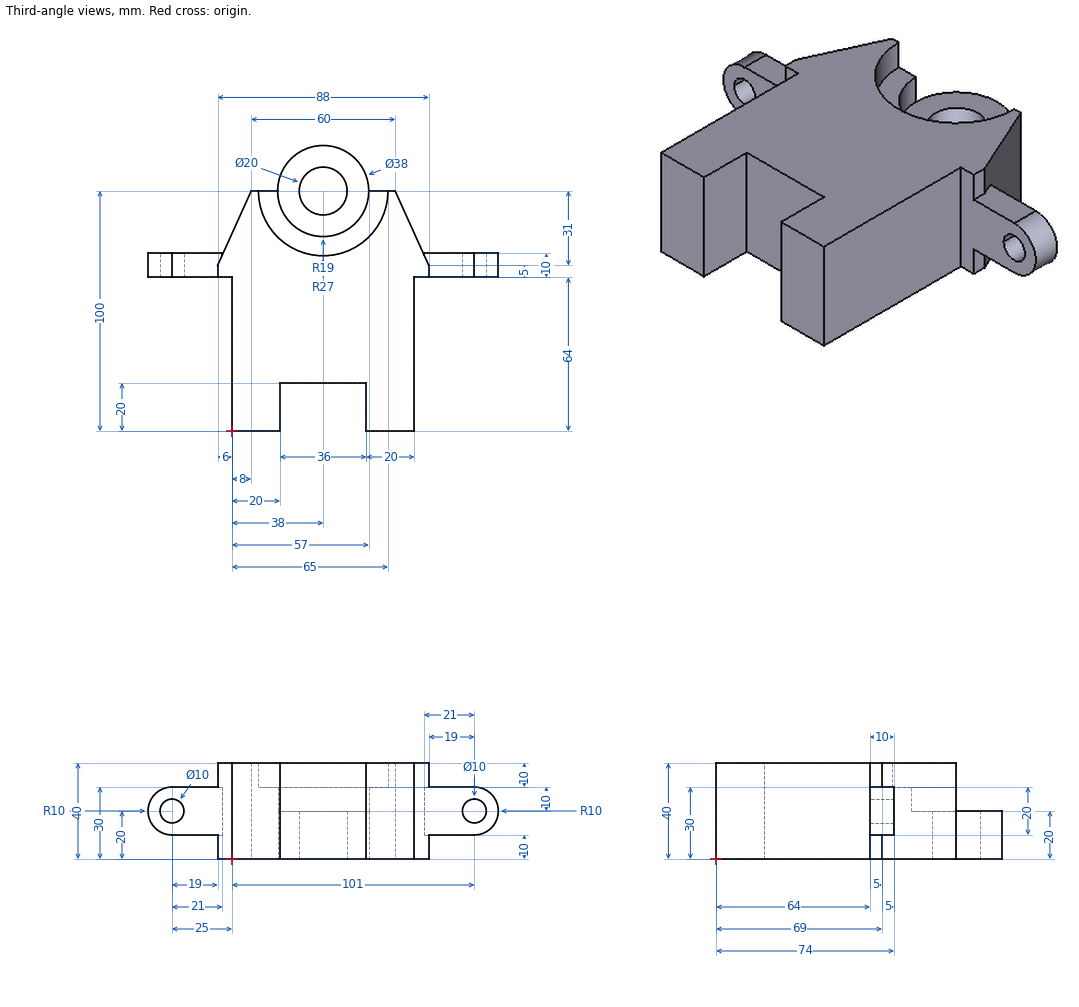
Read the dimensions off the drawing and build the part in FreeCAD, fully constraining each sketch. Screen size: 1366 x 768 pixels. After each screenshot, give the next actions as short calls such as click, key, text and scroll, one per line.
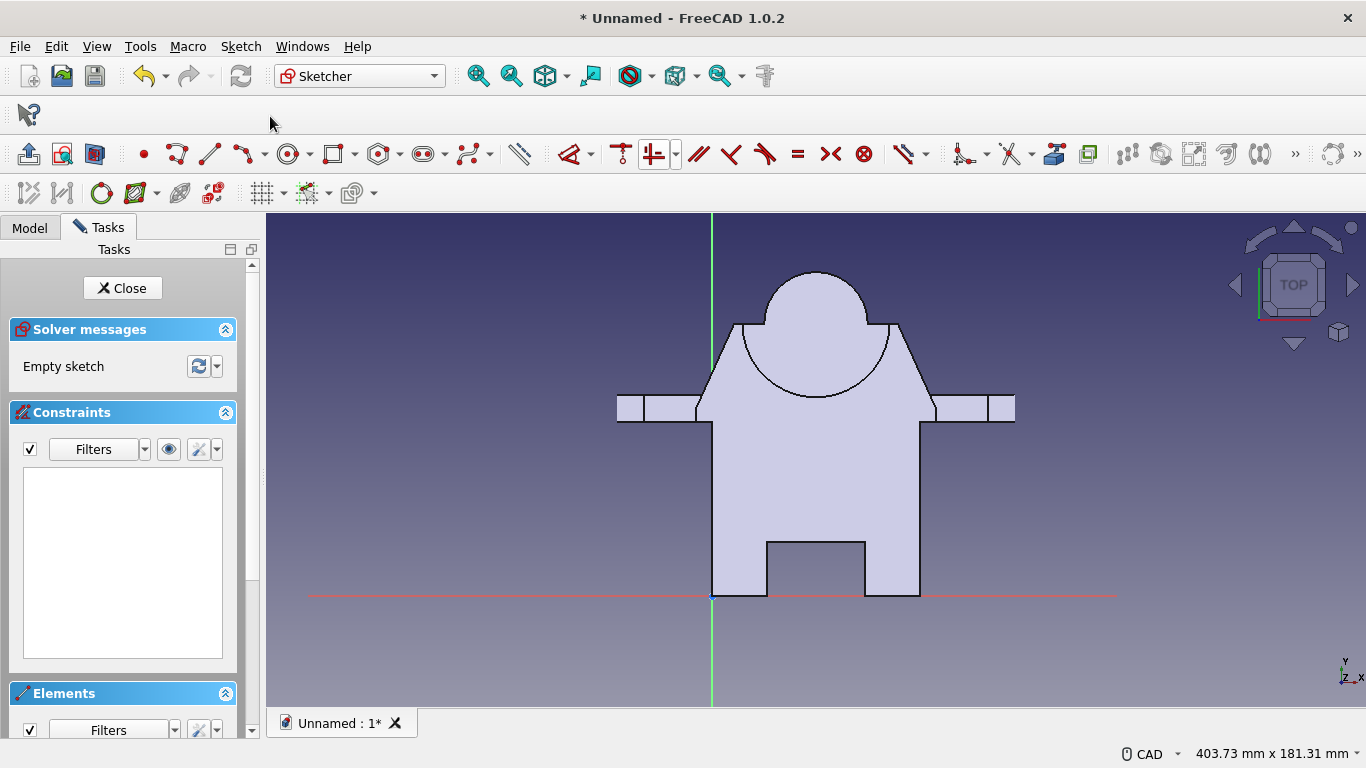
scroll(856, 244, up, 5)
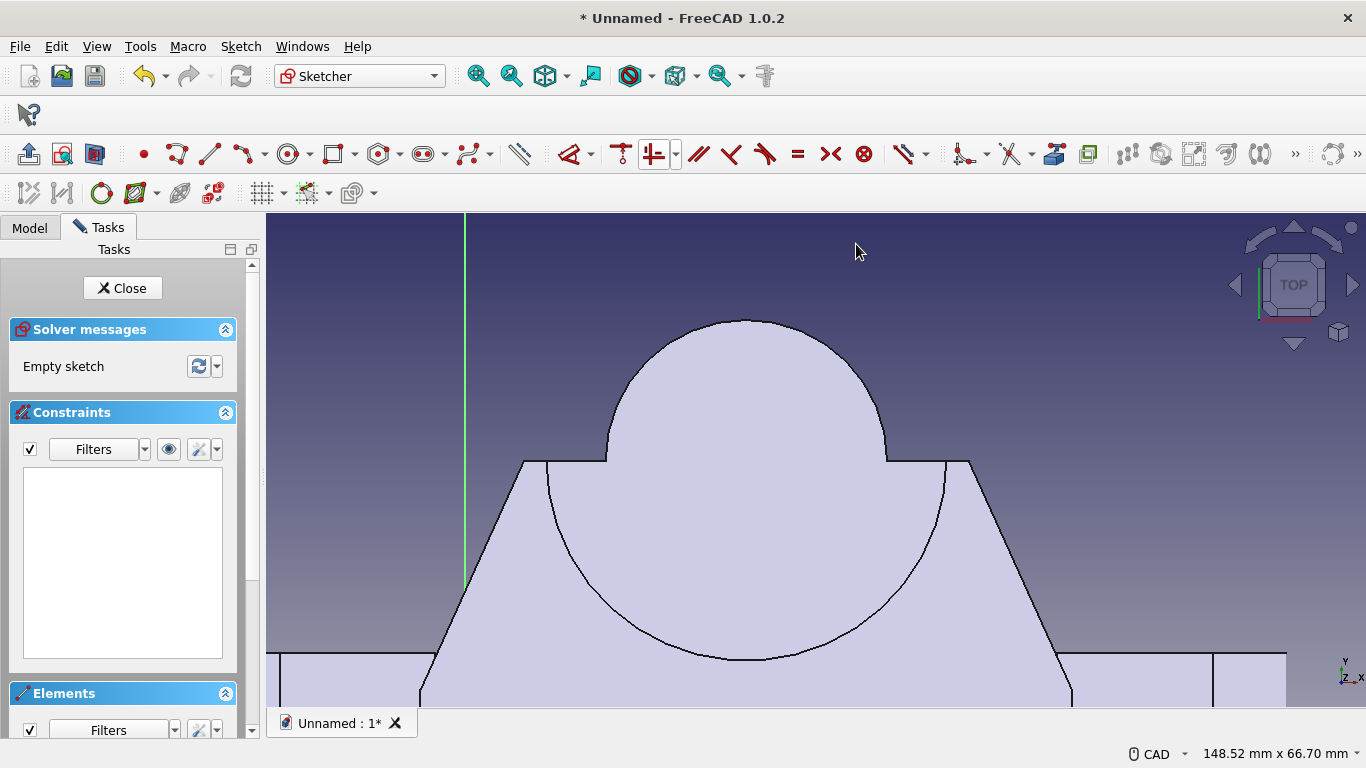
click(288, 154)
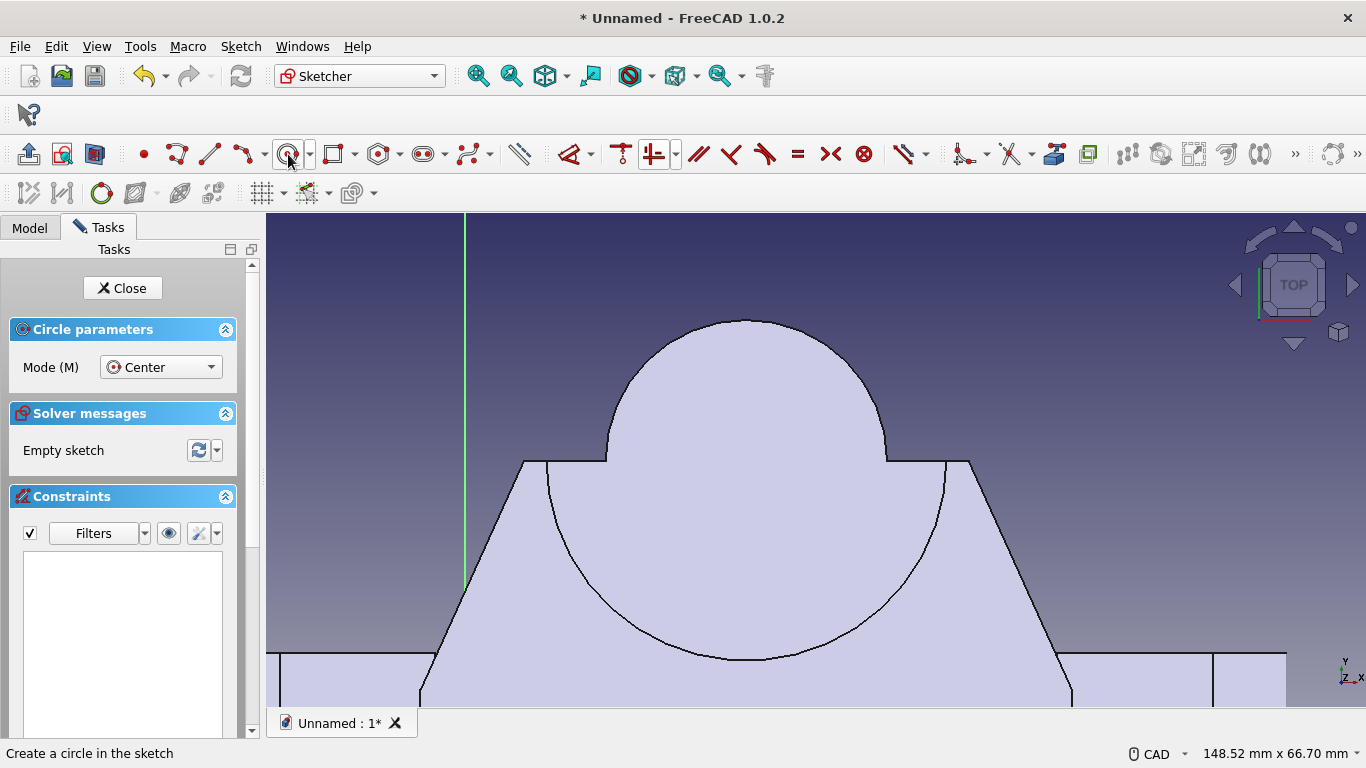
click(746, 461)
click(846, 361)
key(Escape)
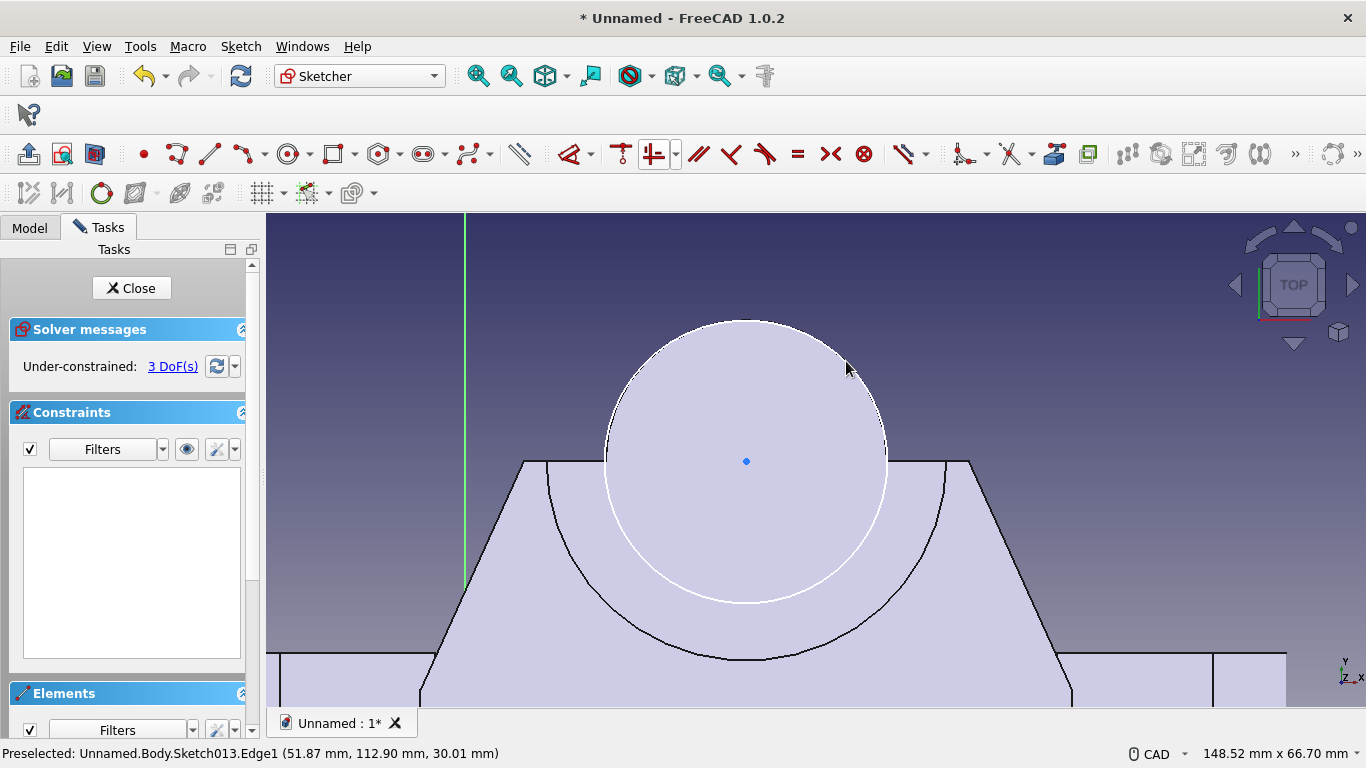
click(568, 154)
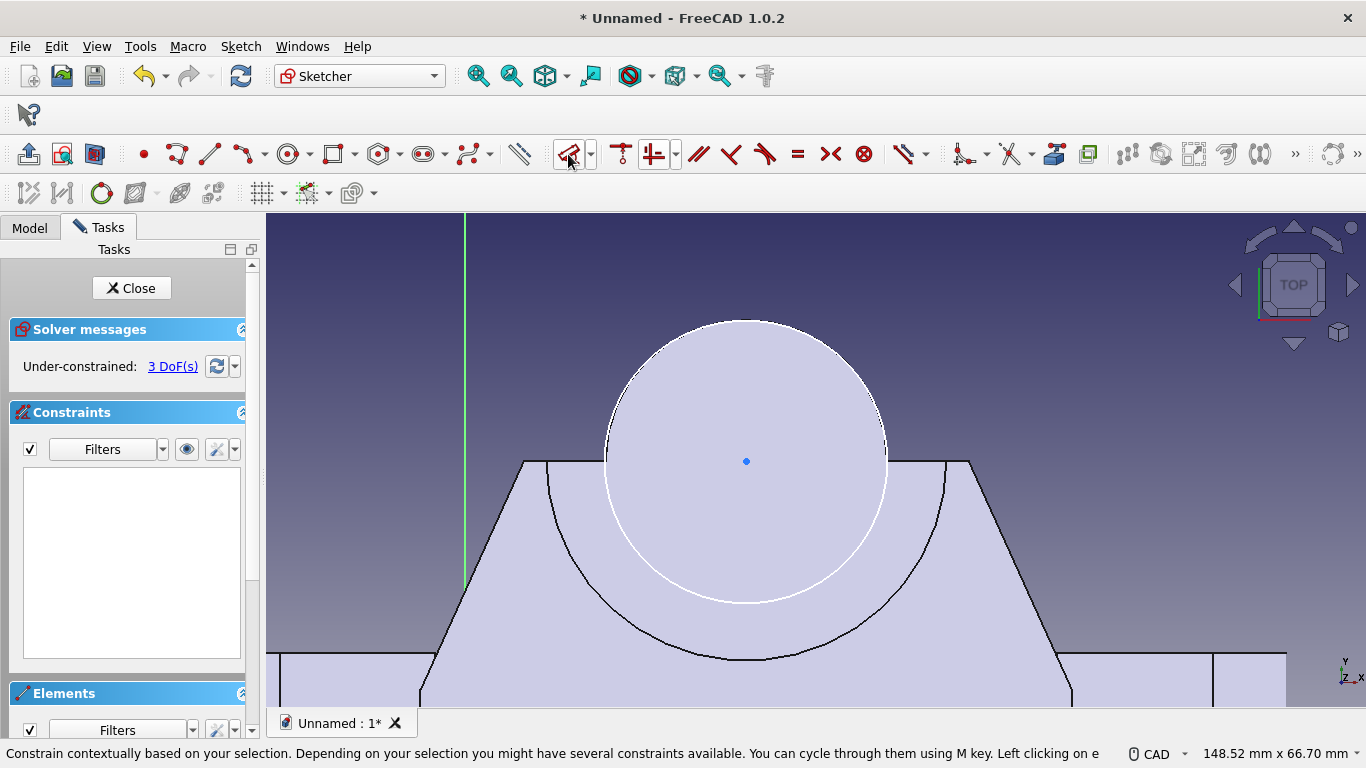
click(846, 362)
click(869, 339)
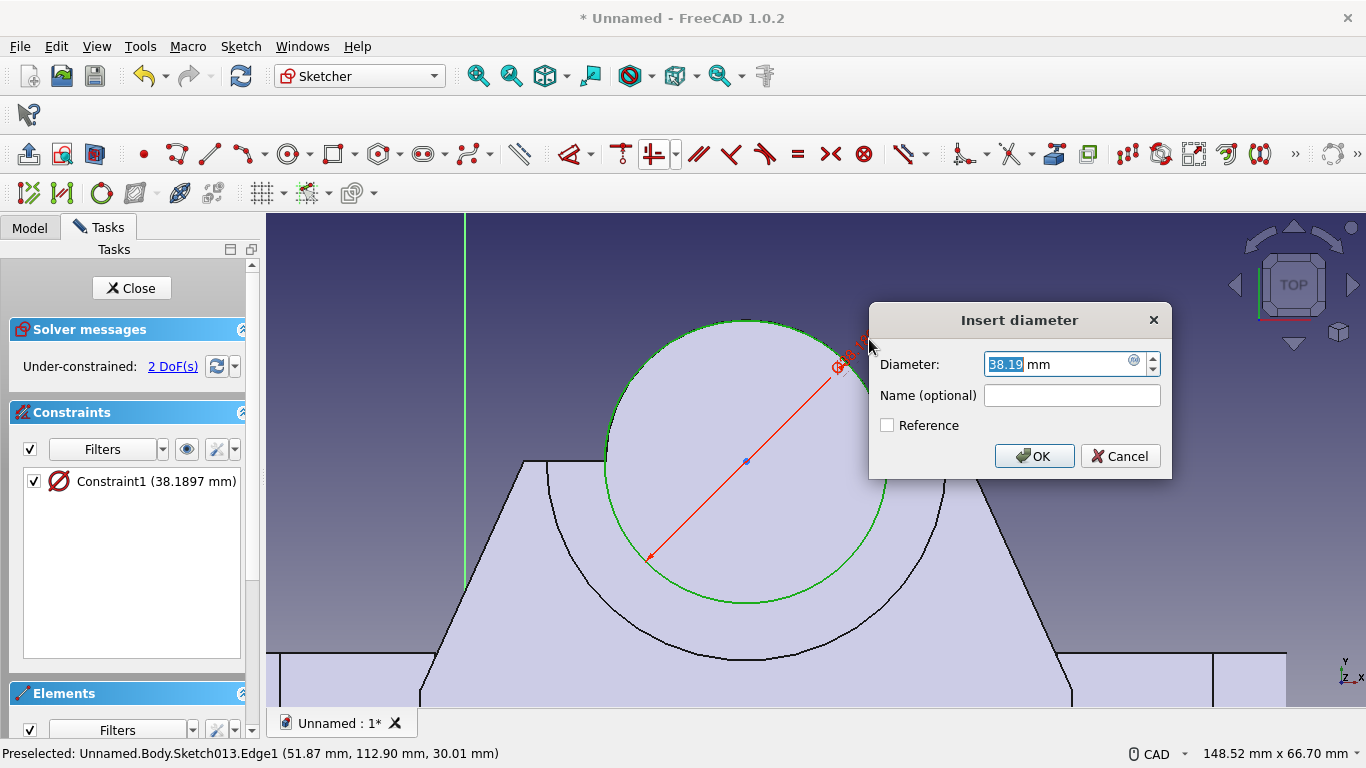
text(38)
key(Return)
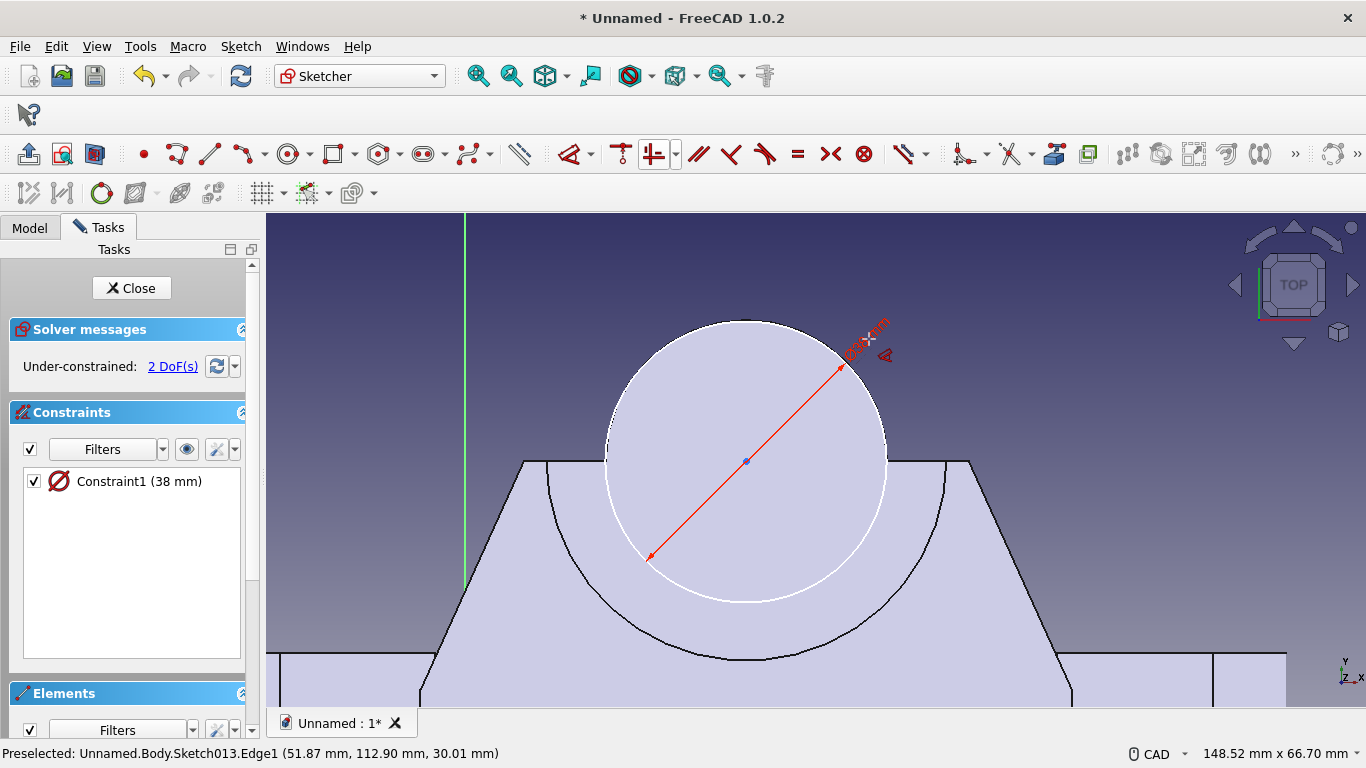
click(746, 462)
click(541, 428)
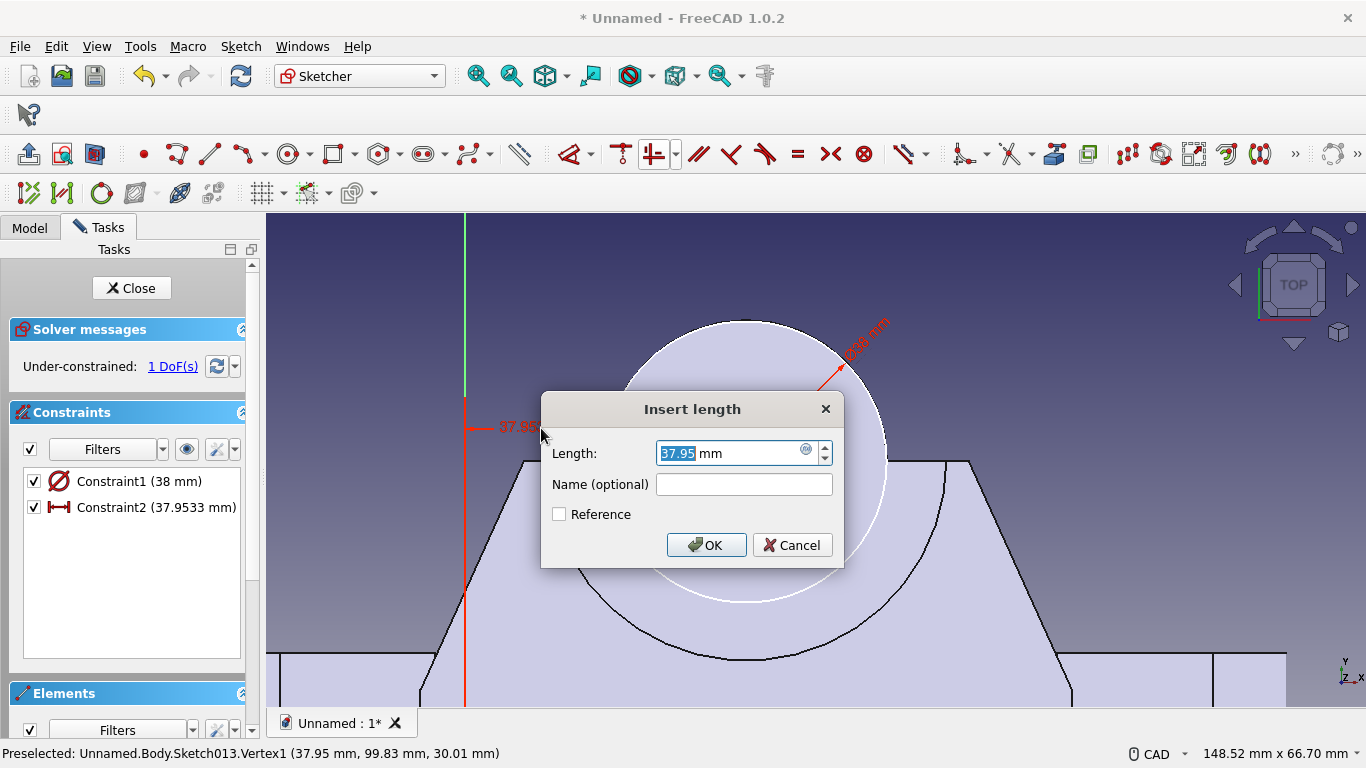
text(38)
key(Return)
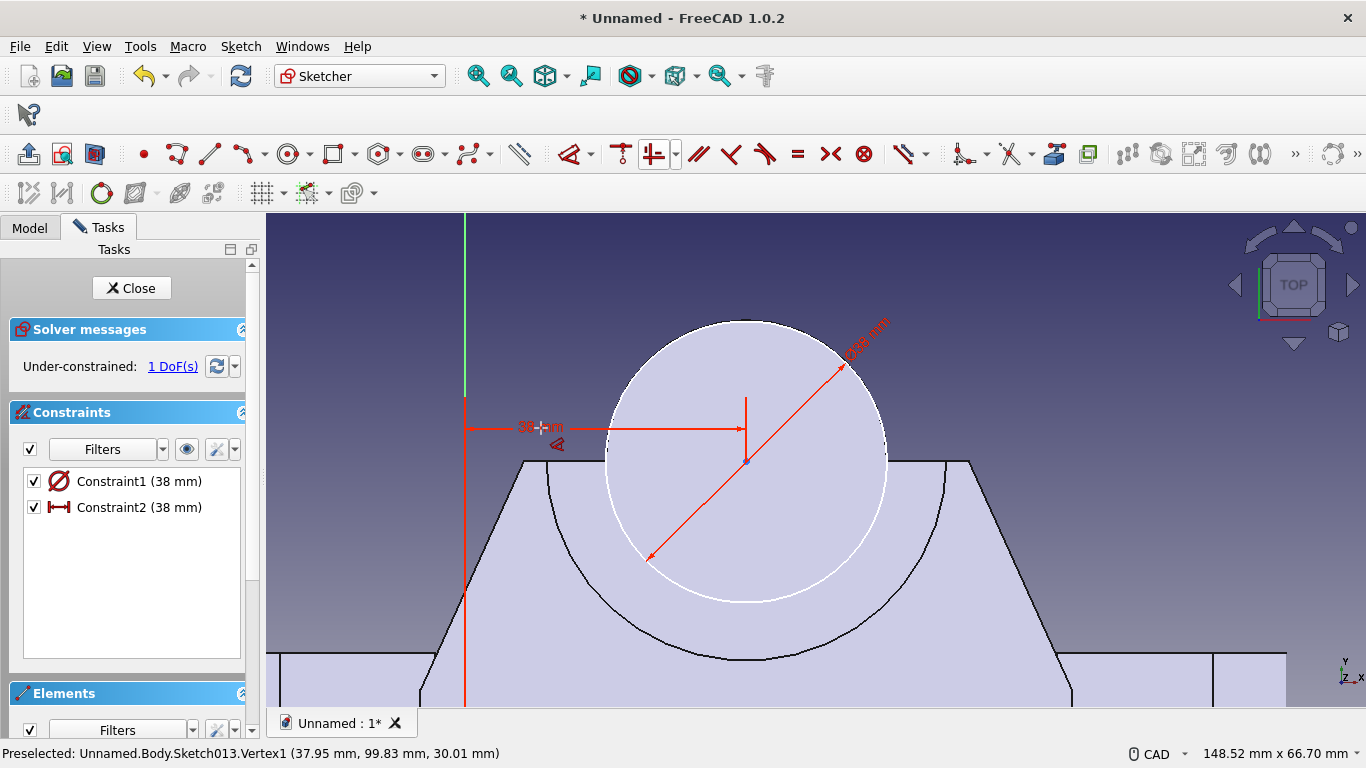
click(746, 462)
click(431, 571)